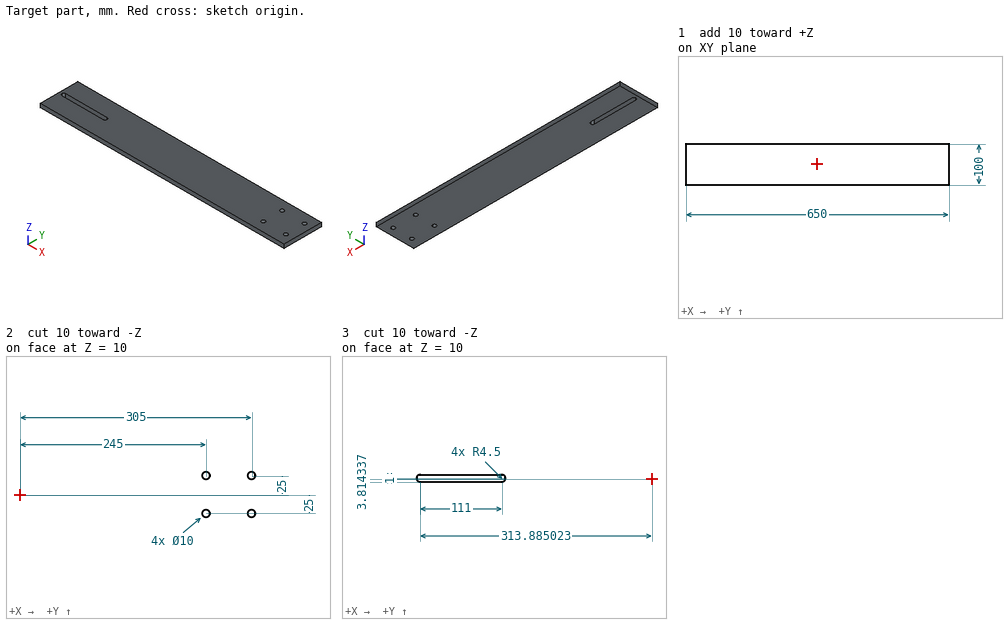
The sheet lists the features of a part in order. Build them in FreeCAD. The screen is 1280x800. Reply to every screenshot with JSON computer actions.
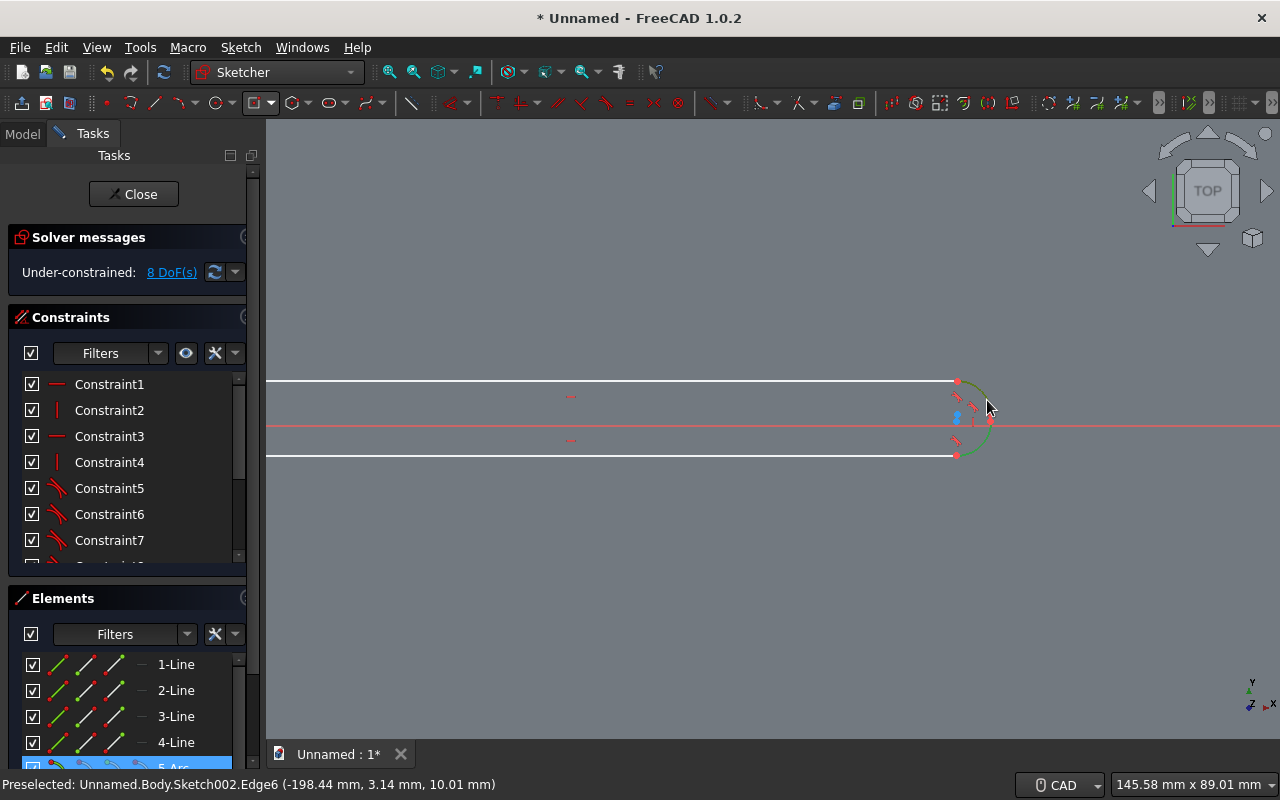
{"action": "scroll", "coordinate": [974, 451], "scroll_direction": "down", "scroll_amount": 2}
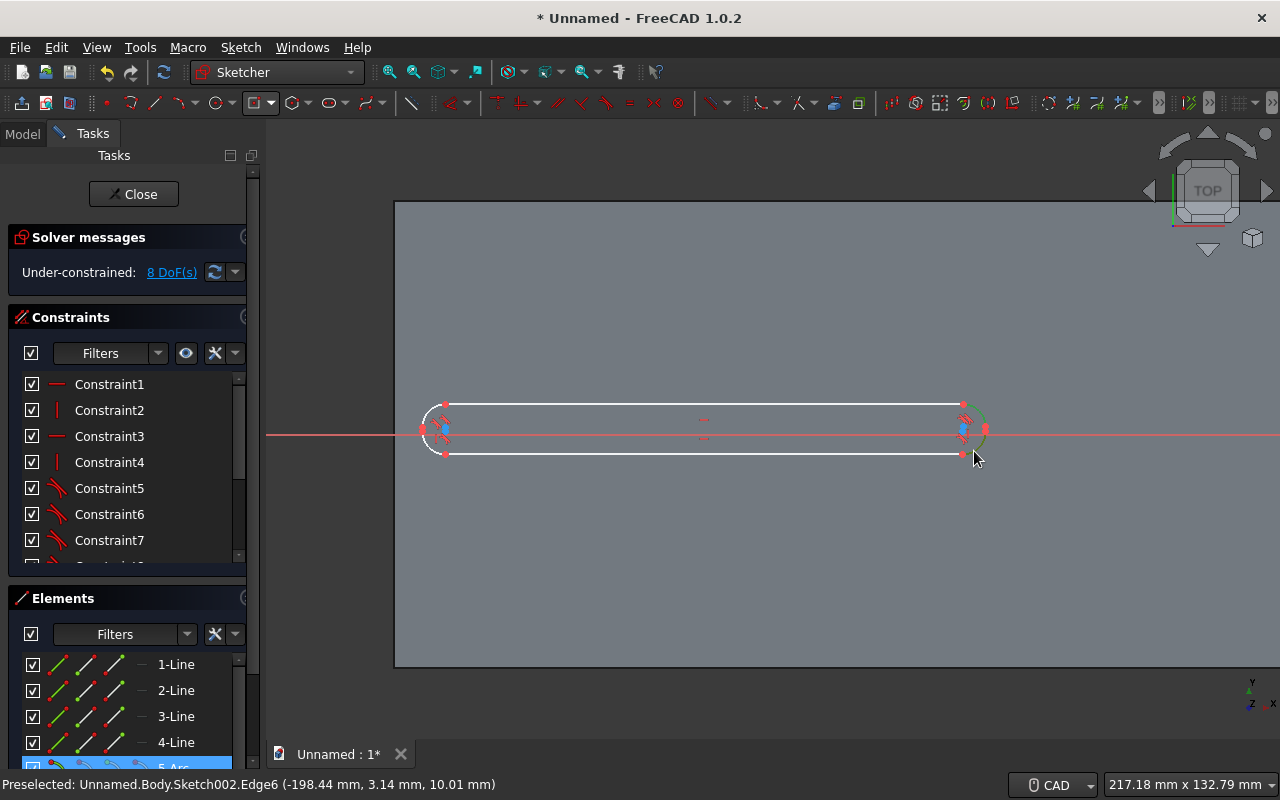
{"action": "scroll", "coordinate": [435, 407], "scroll_direction": "up", "scroll_amount": 2}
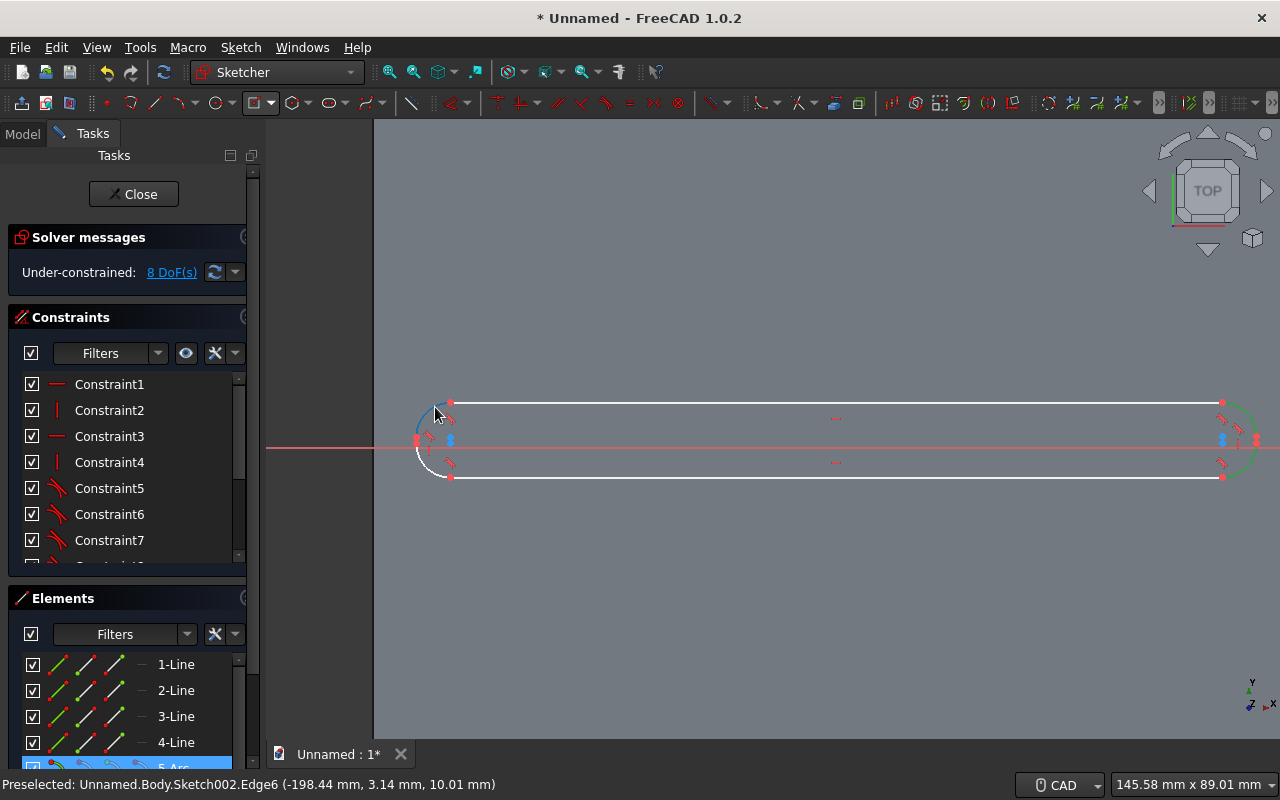
{"action": "left_click", "coordinate": [435, 407]}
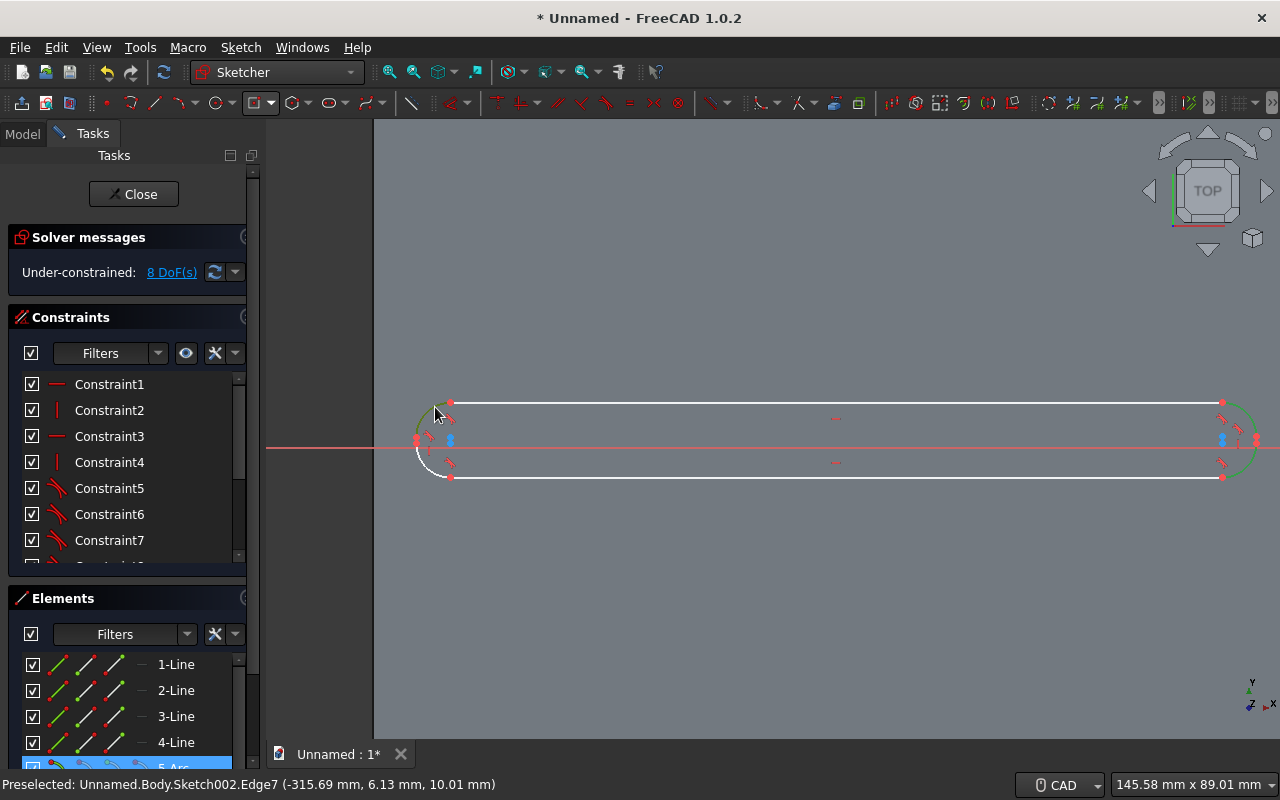
{"action": "scroll", "coordinate": [420, 459], "scroll_direction": "up", "scroll_amount": 2}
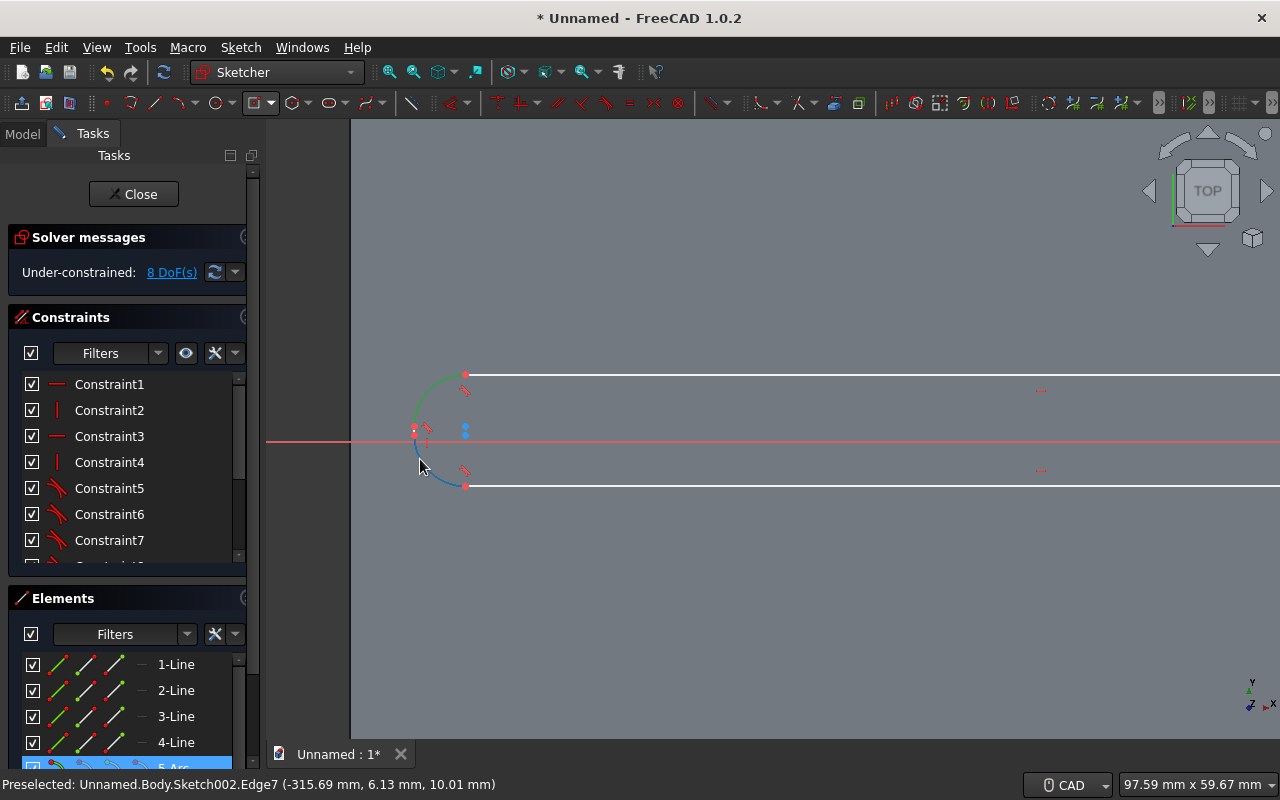
{"action": "left_click", "coordinate": [420, 459]}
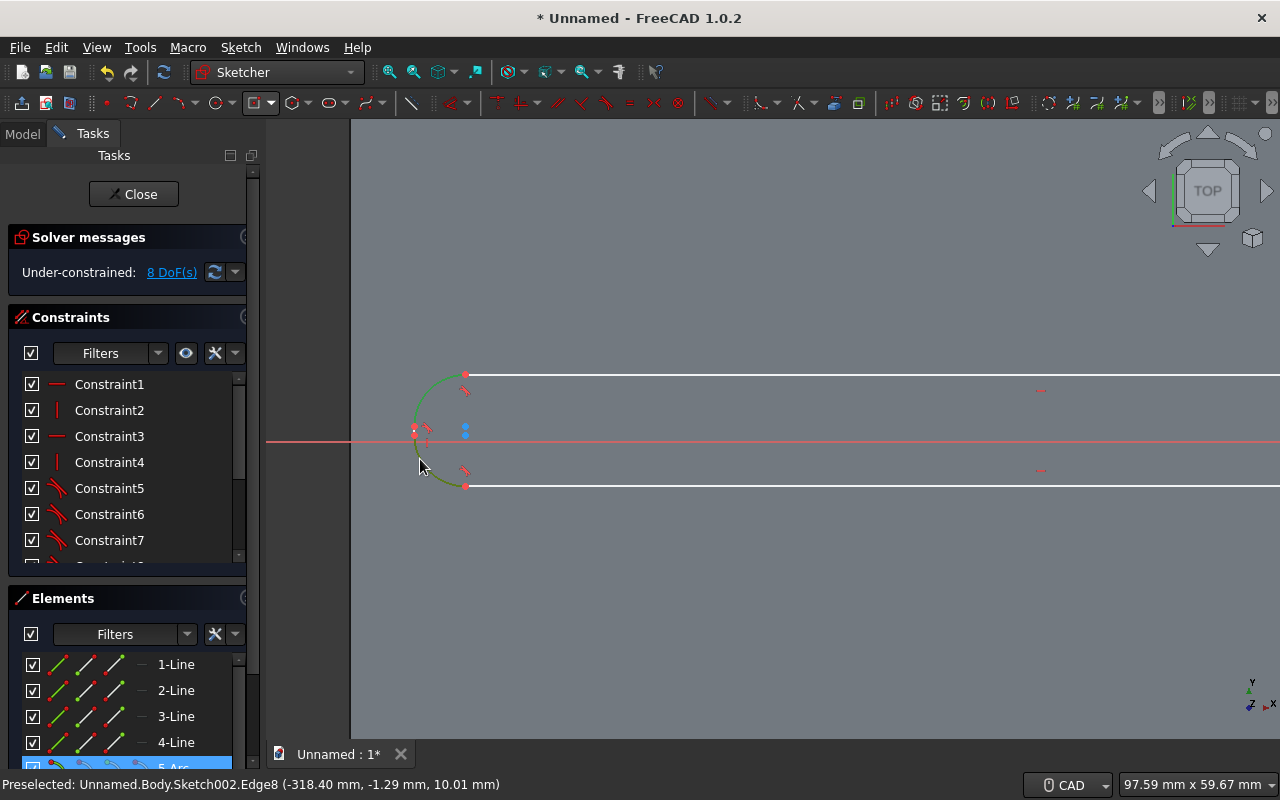
{"action": "key", "text": "e"}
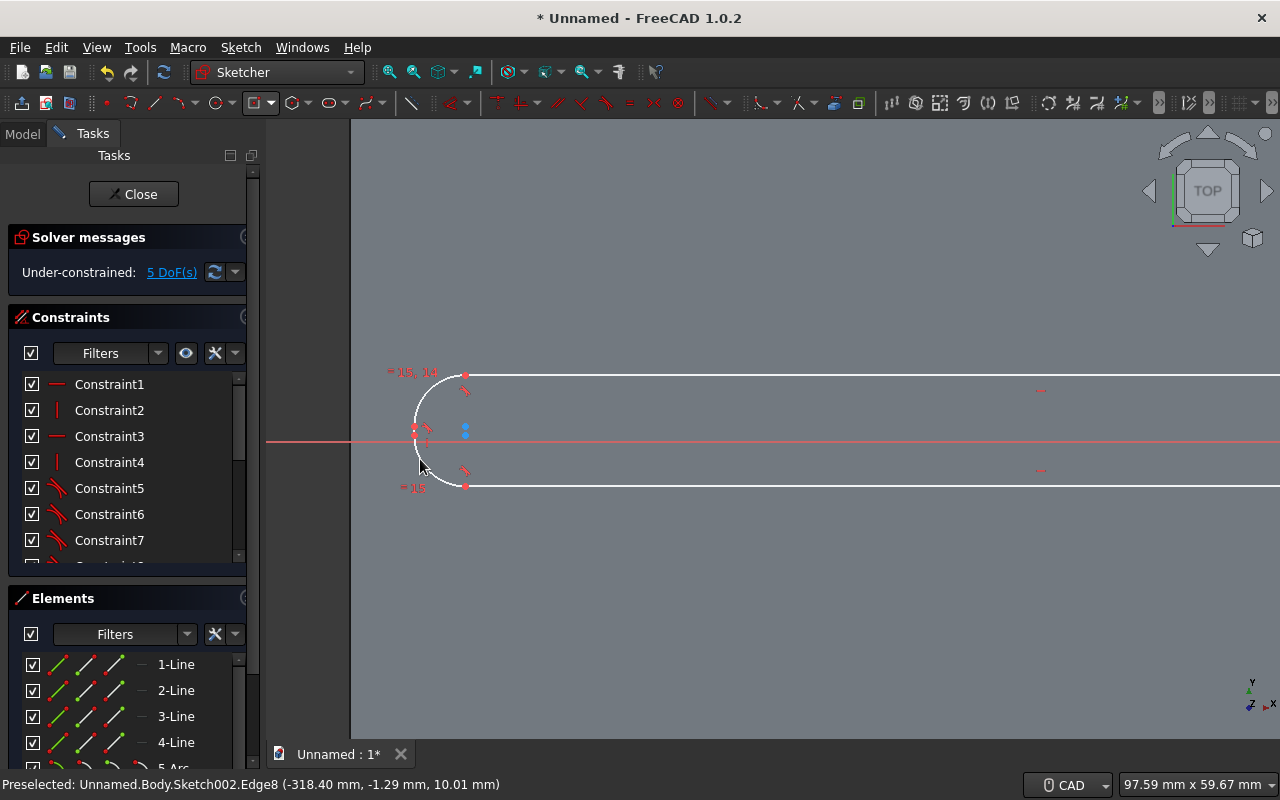
{"action": "left_click", "coordinate": [450, 104]}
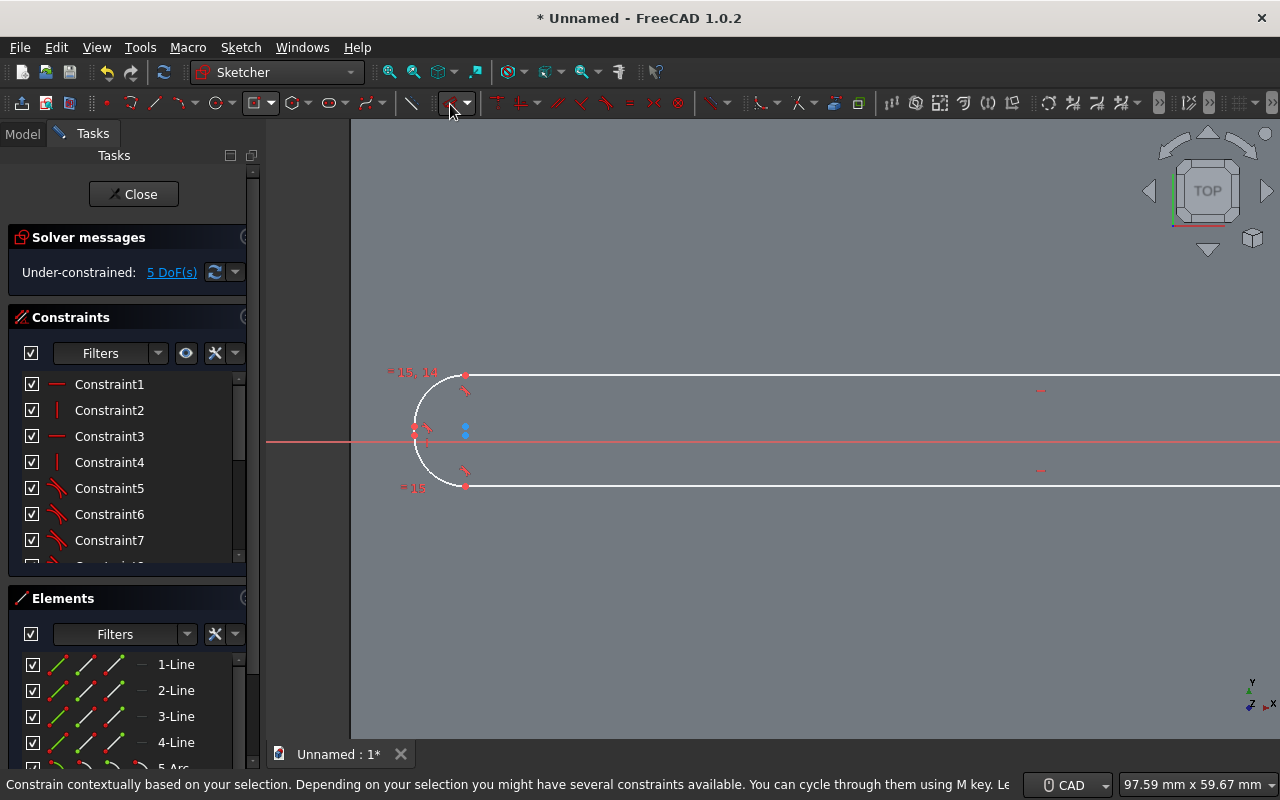
{"action": "scroll", "coordinate": [429, 428], "scroll_direction": "down", "scroll_amount": 4}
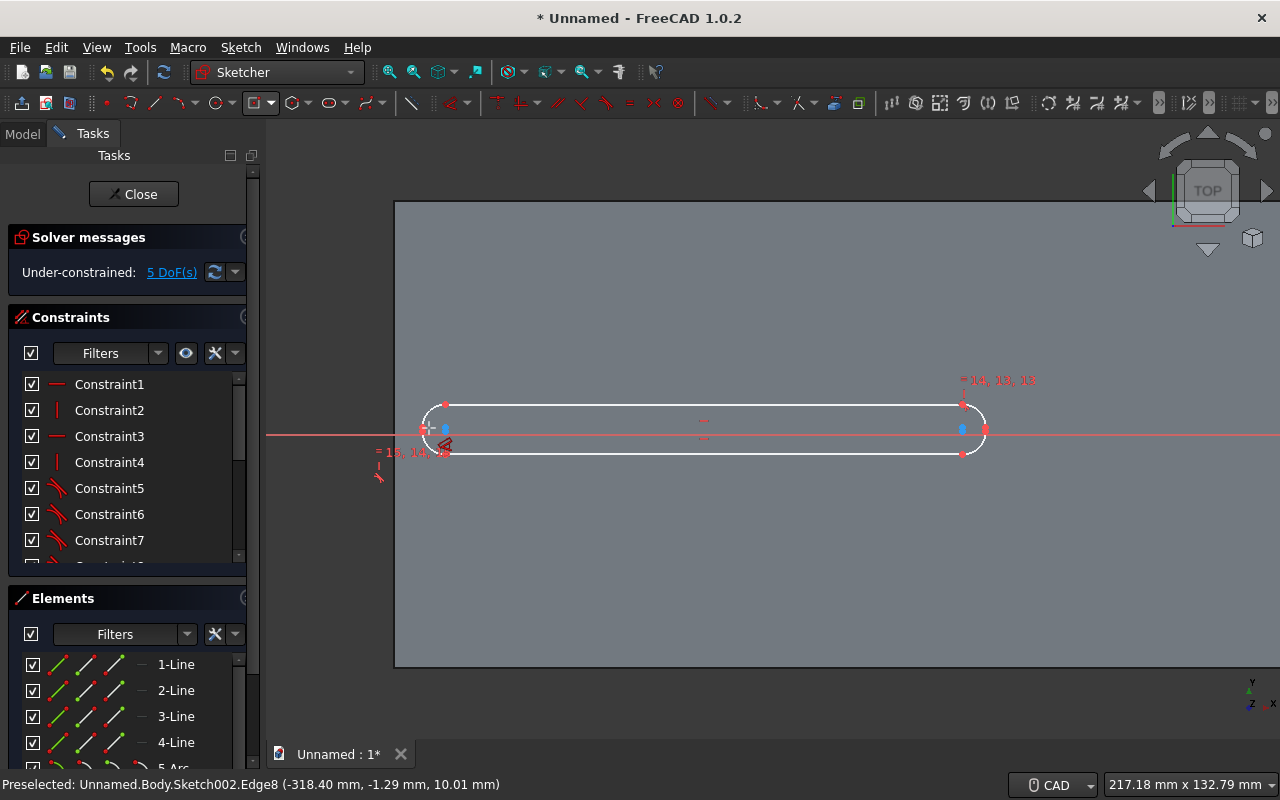
{"action": "scroll", "coordinate": [973, 452], "scroll_direction": "up", "scroll_amount": 4}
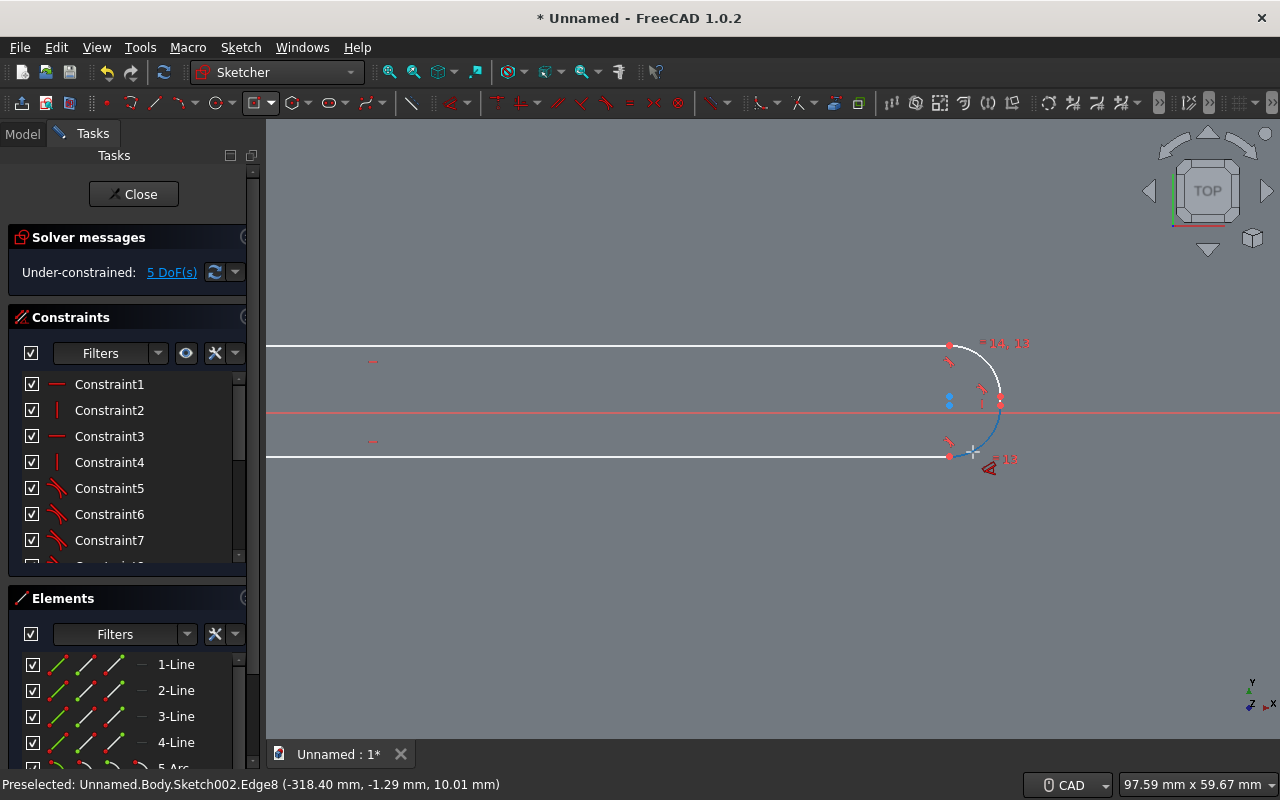
{"action": "left_click", "coordinate": [973, 451]}
{"action": "left_click", "coordinate": [988, 479]}